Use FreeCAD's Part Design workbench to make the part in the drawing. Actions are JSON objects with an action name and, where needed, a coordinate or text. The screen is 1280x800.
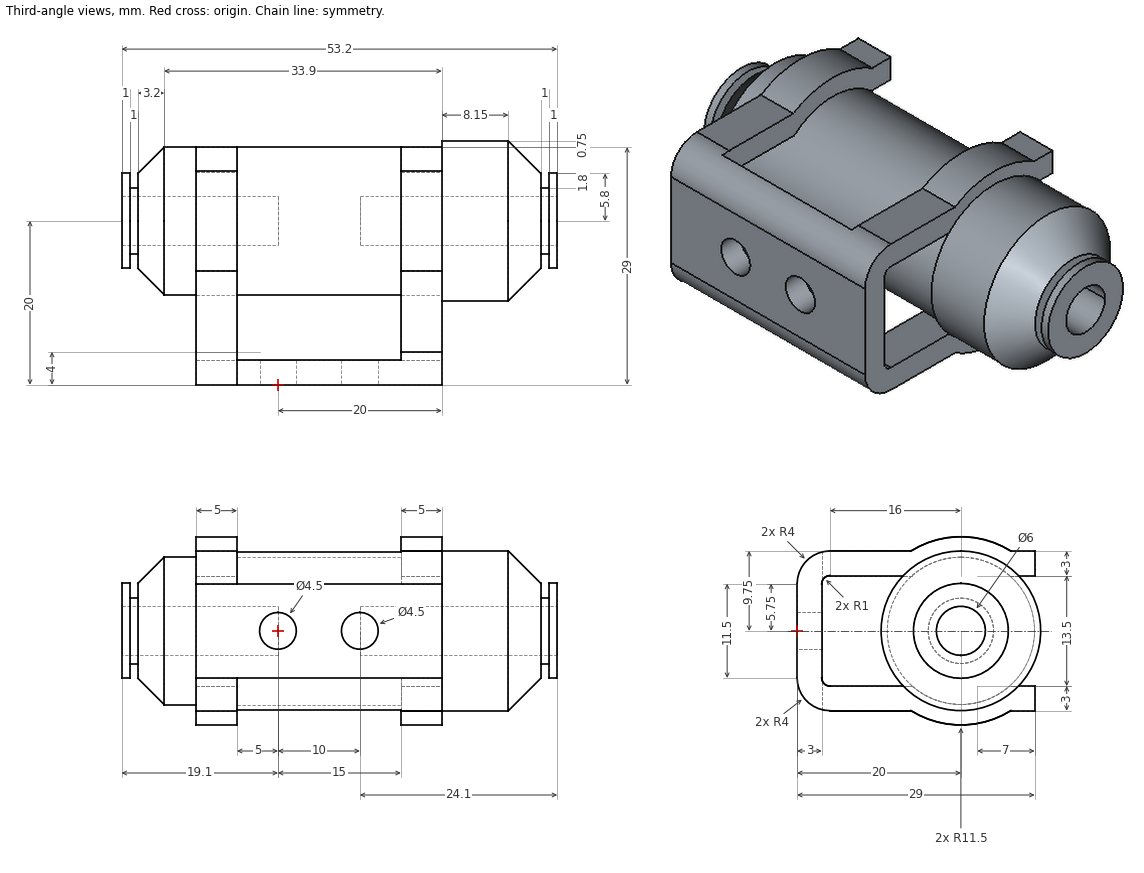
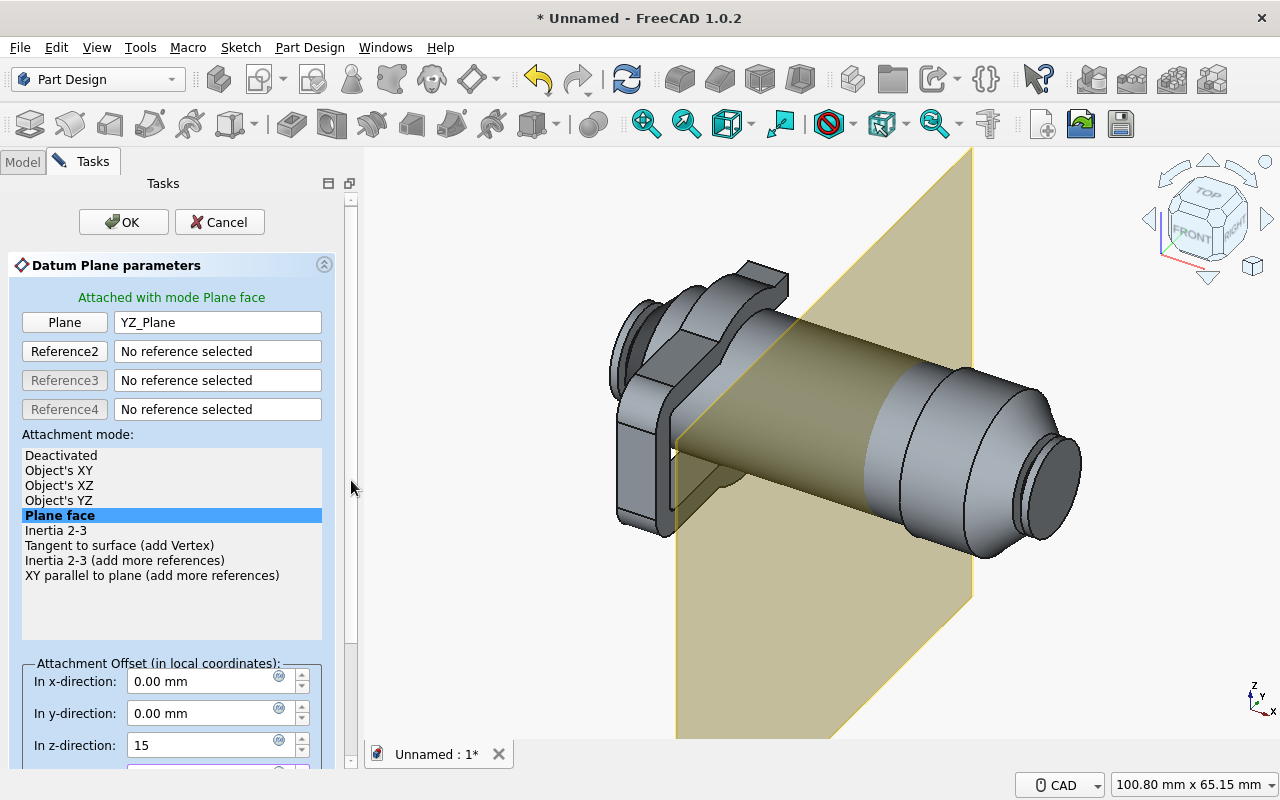
{"action": "left_click", "coordinate": [124, 222]}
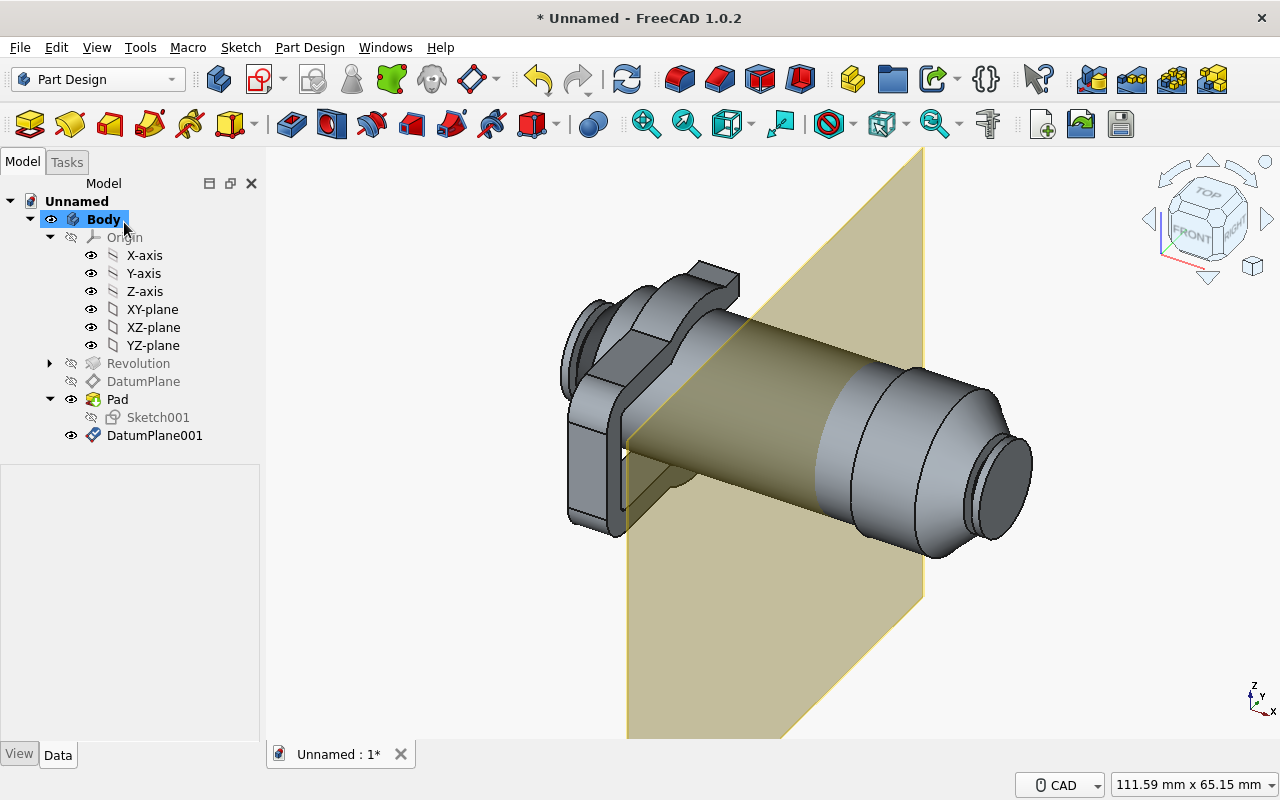
{"action": "left_click", "coordinate": [116, 435]}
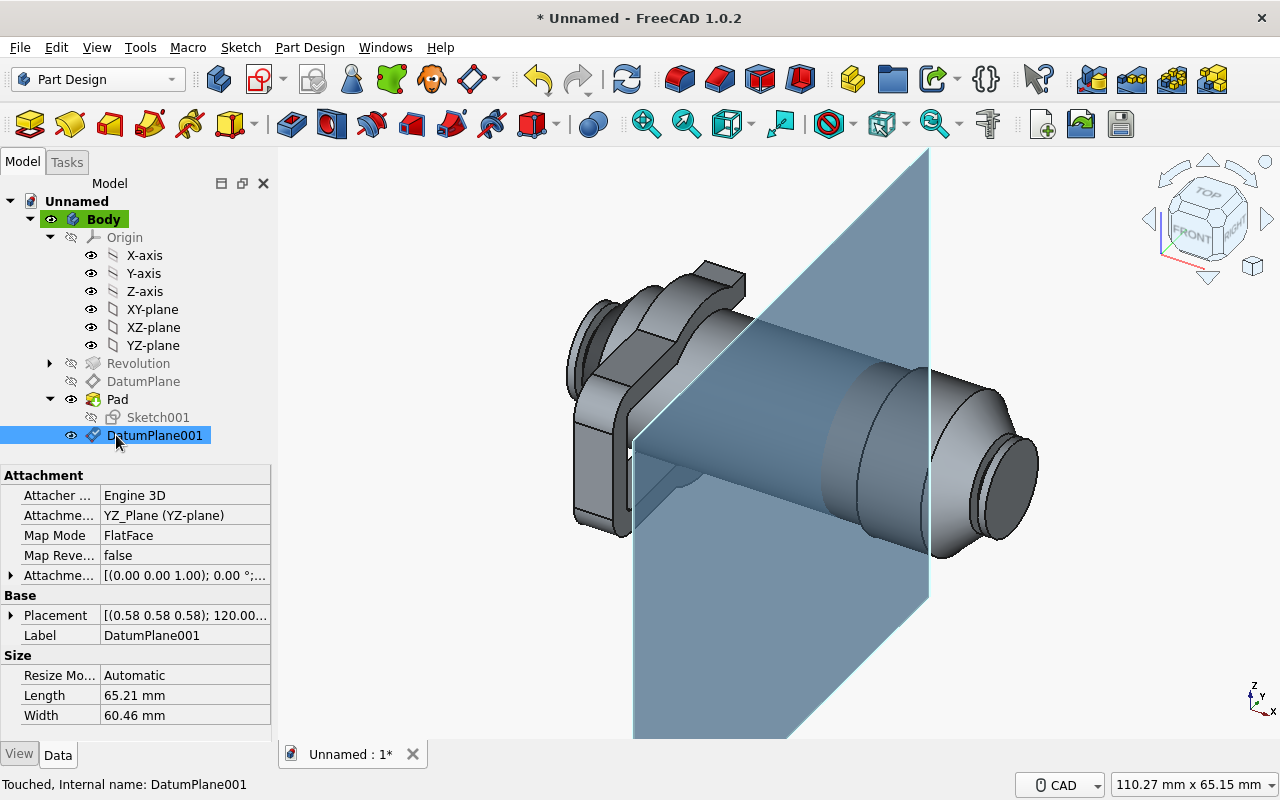
{"action": "left_click", "coordinate": [260, 80]}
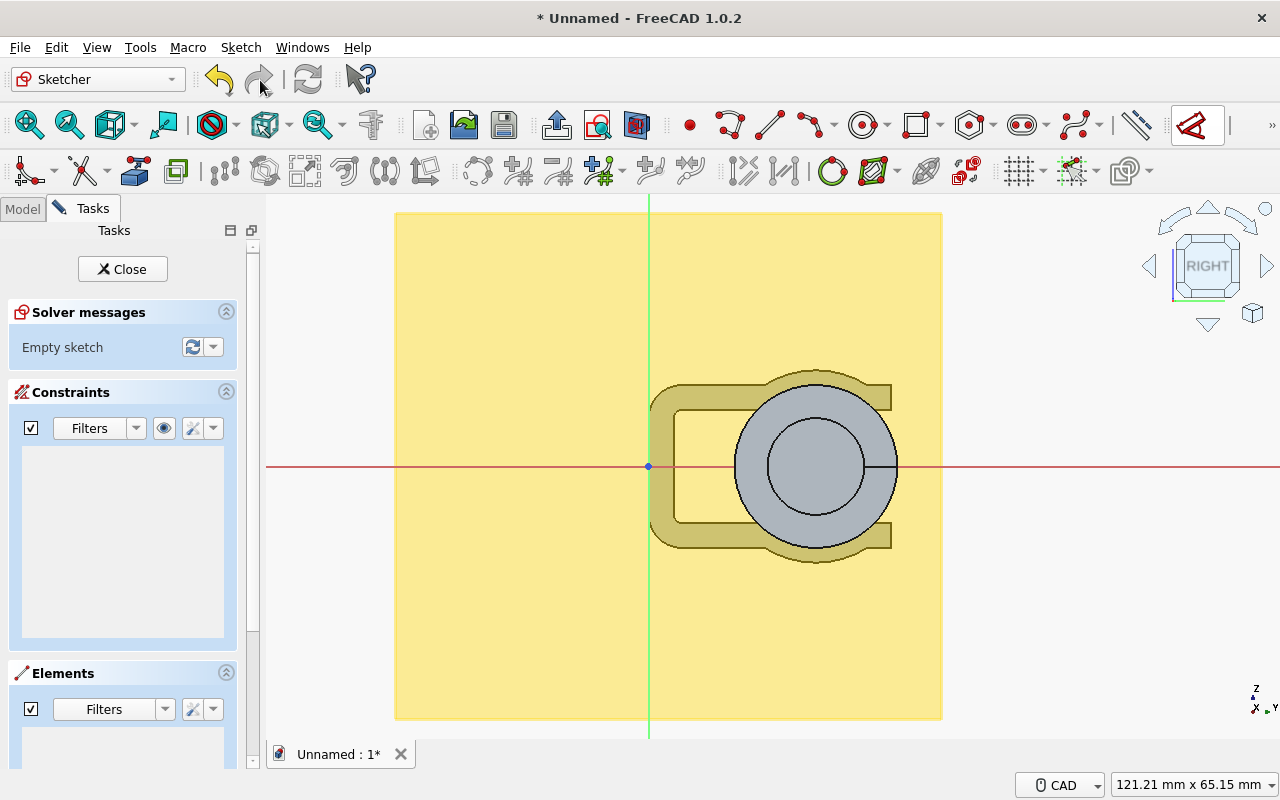
{"action": "left_click", "coordinate": [638, 126]}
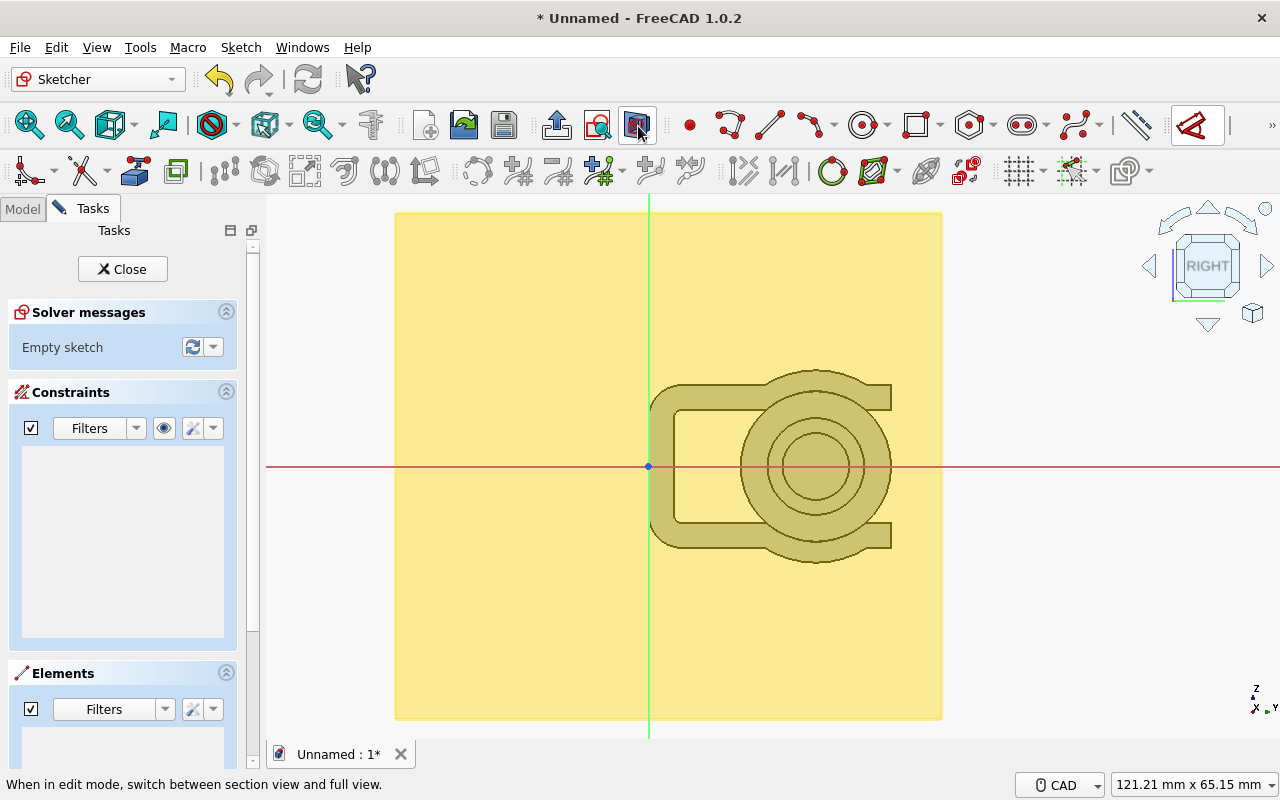
{"action": "scroll", "coordinate": [849, 466], "scroll_direction": "up", "scroll_amount": 3}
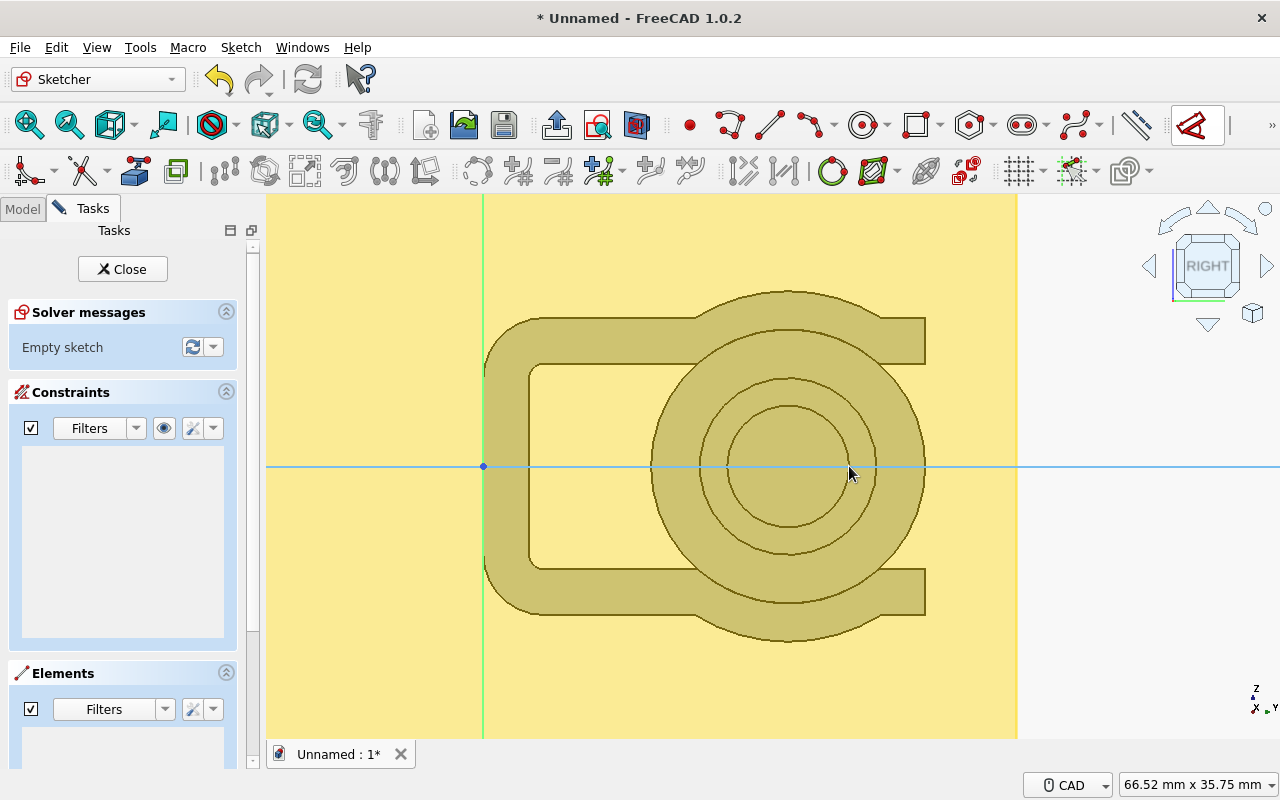
{"action": "left_click", "coordinate": [770, 126]}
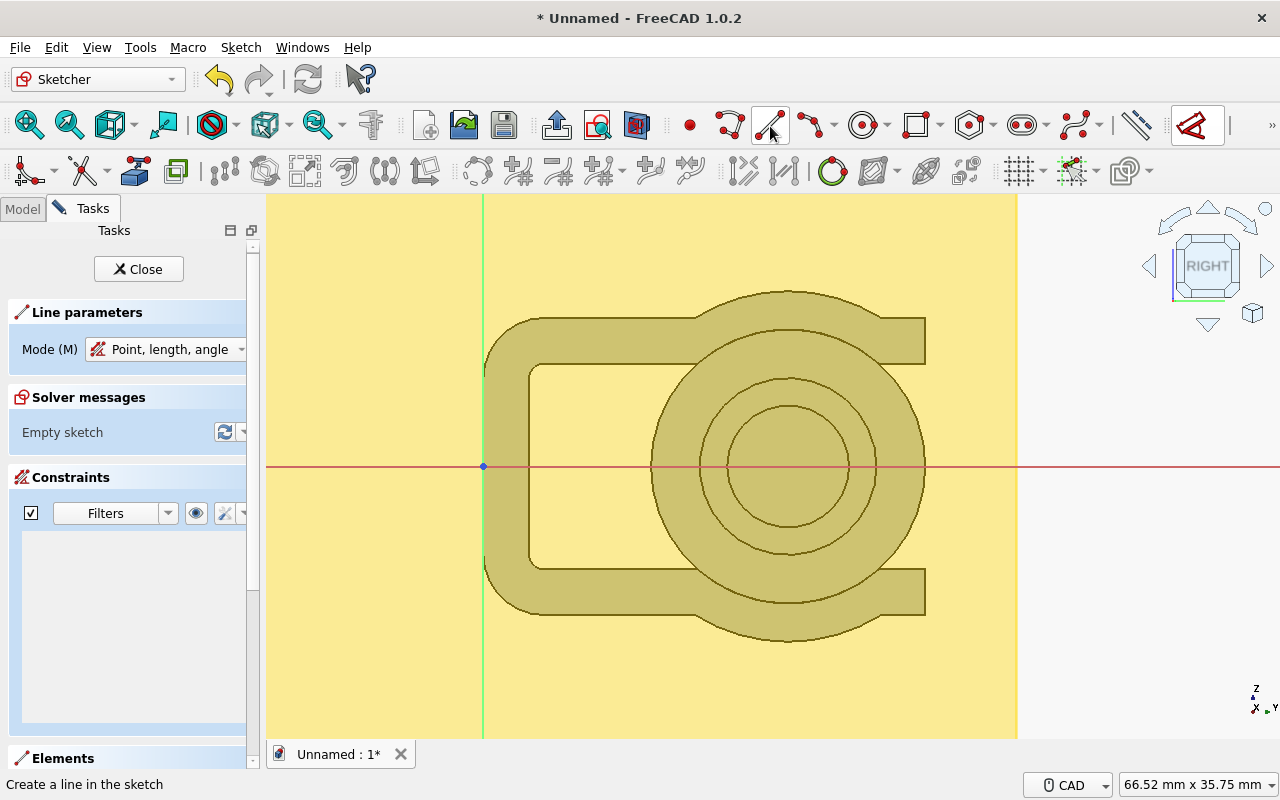
{"action": "left_click", "coordinate": [695, 318]}
{"action": "left_click", "coordinate": [544, 318]}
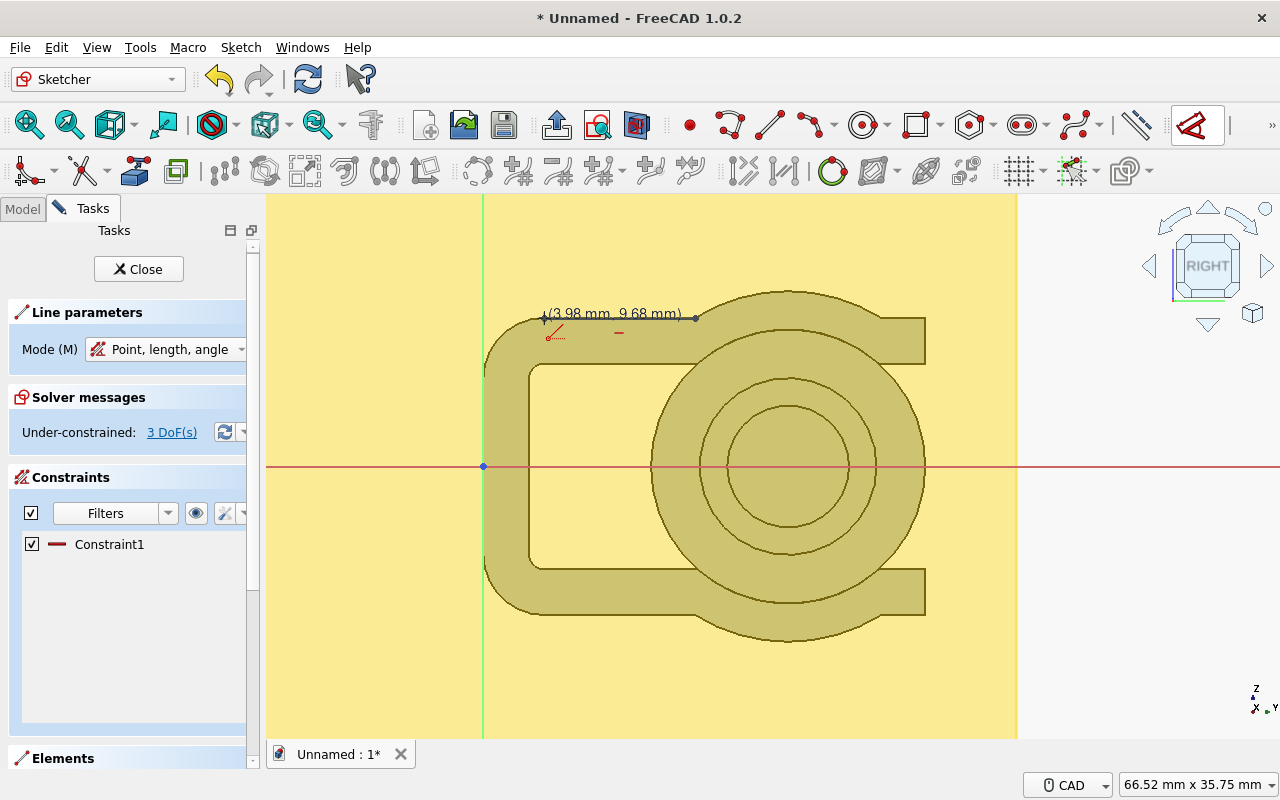
{"action": "left_click", "coordinate": [483, 379]}
{"action": "left_click", "coordinate": [492, 554]}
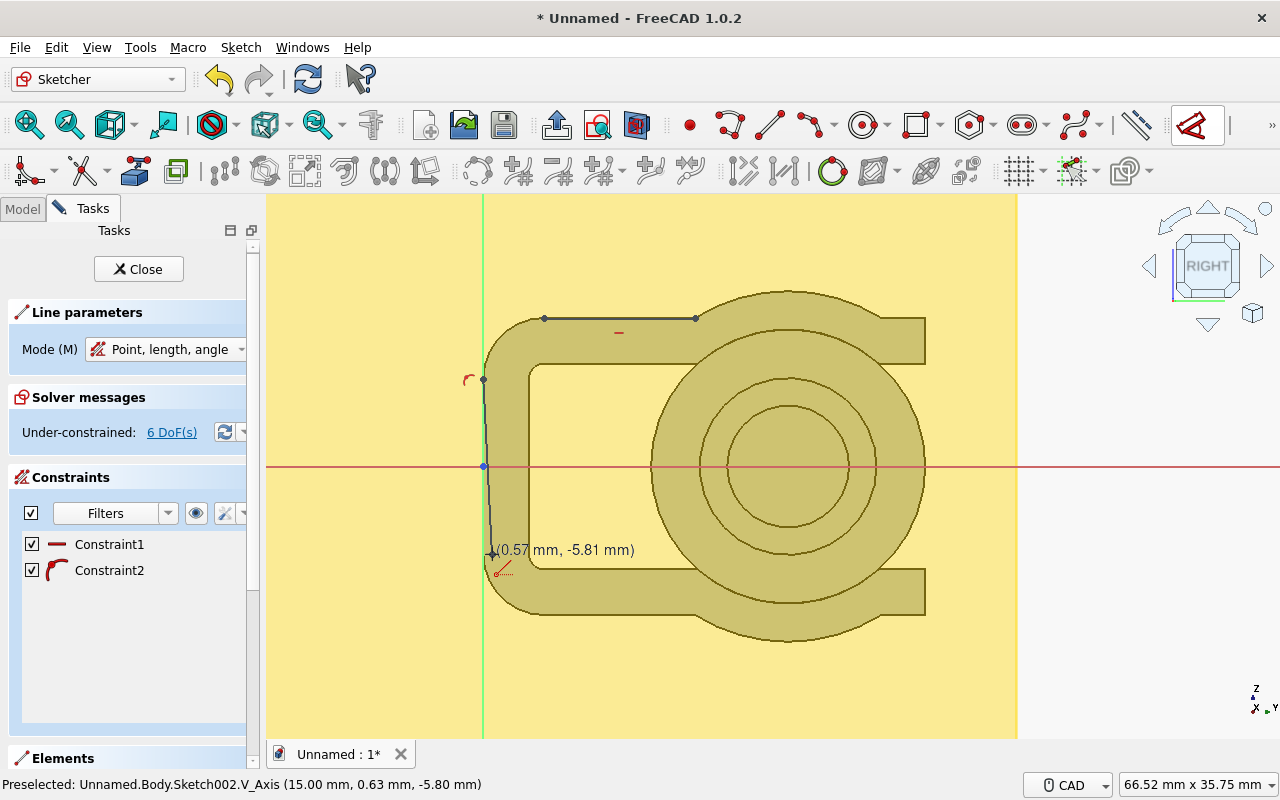
{"action": "left_click", "coordinate": [544, 615]}
{"action": "left_click", "coordinate": [695, 615]}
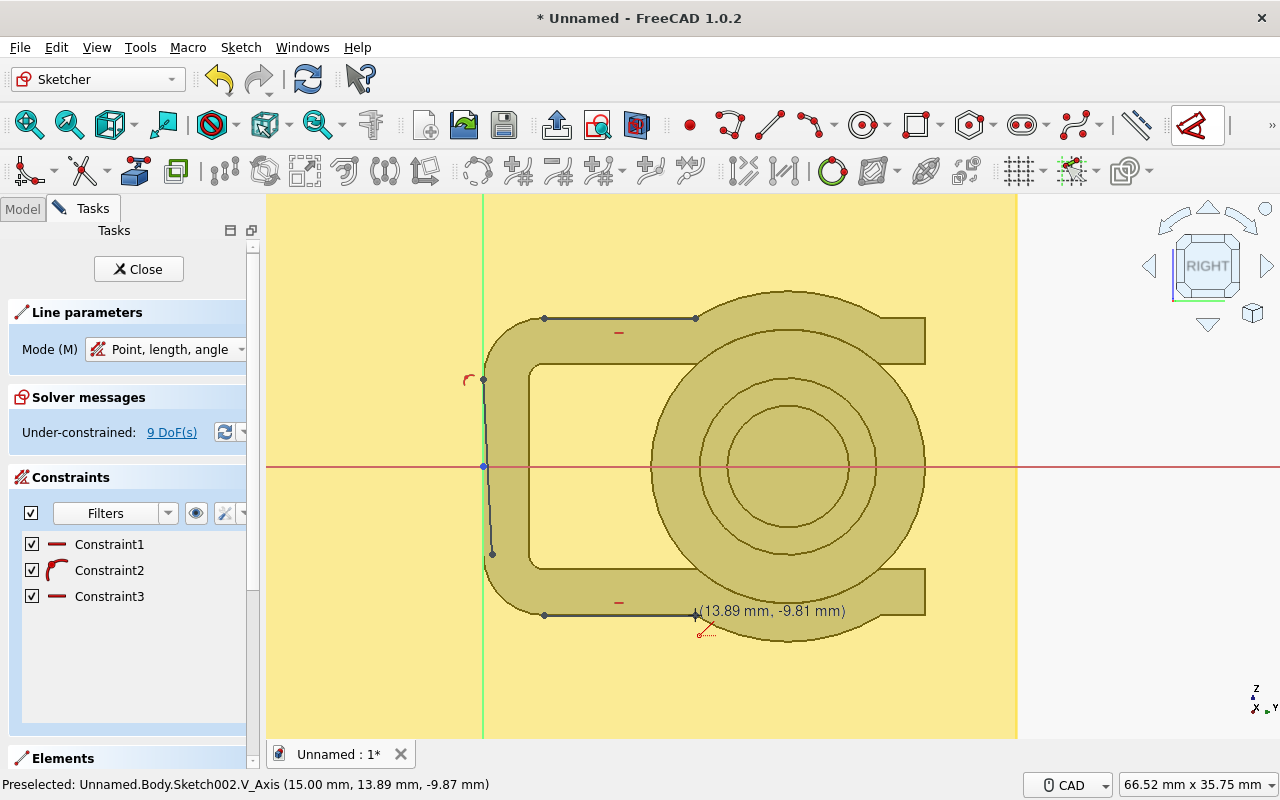
{"action": "left_click", "coordinate": [730, 126]}